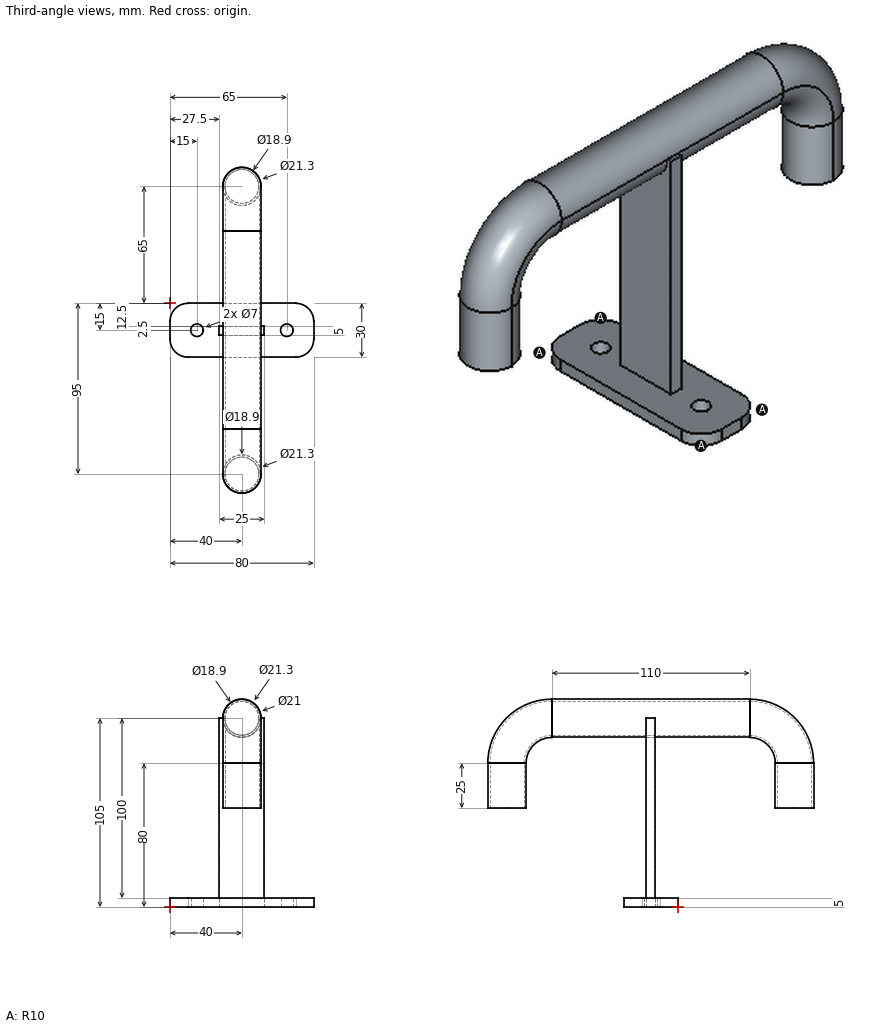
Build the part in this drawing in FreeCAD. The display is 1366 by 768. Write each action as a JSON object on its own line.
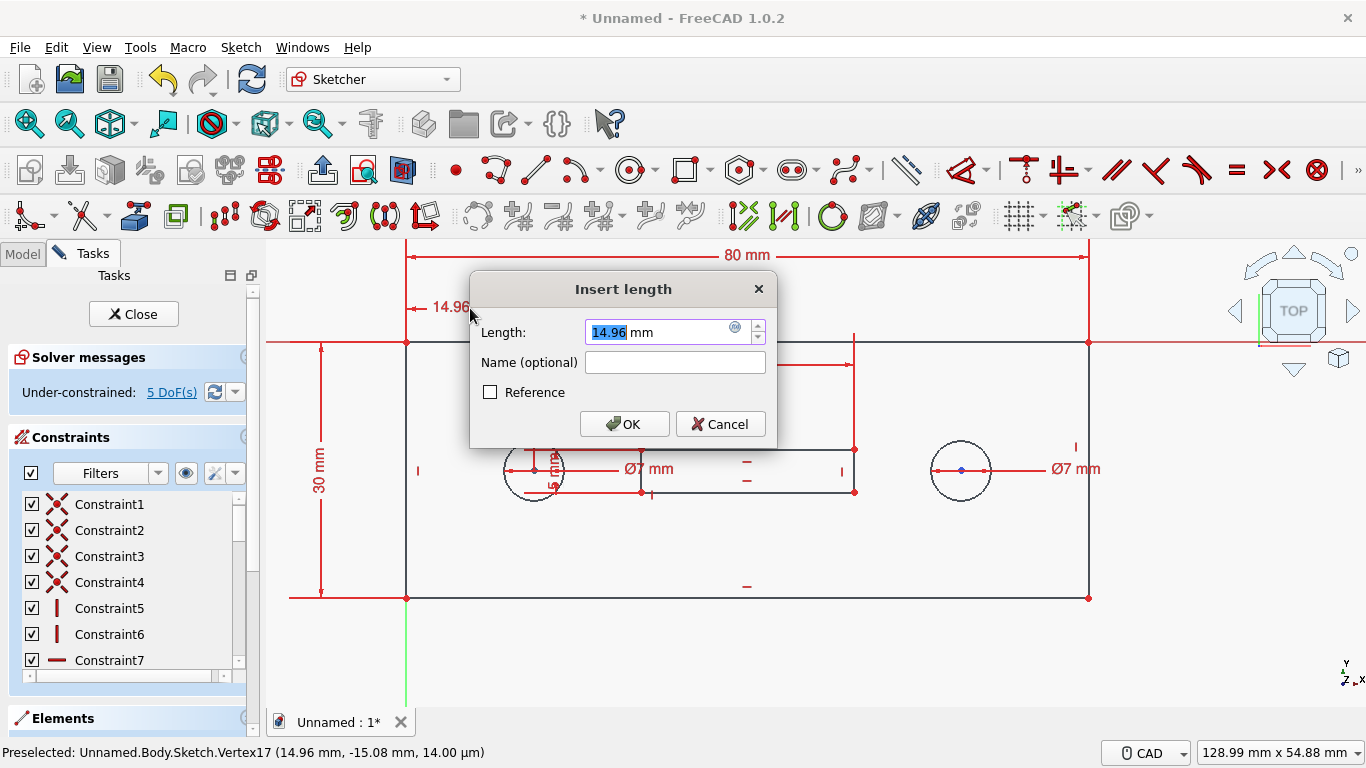
{"action": "type", "text": "15"}
{"action": "key", "text": "Return"}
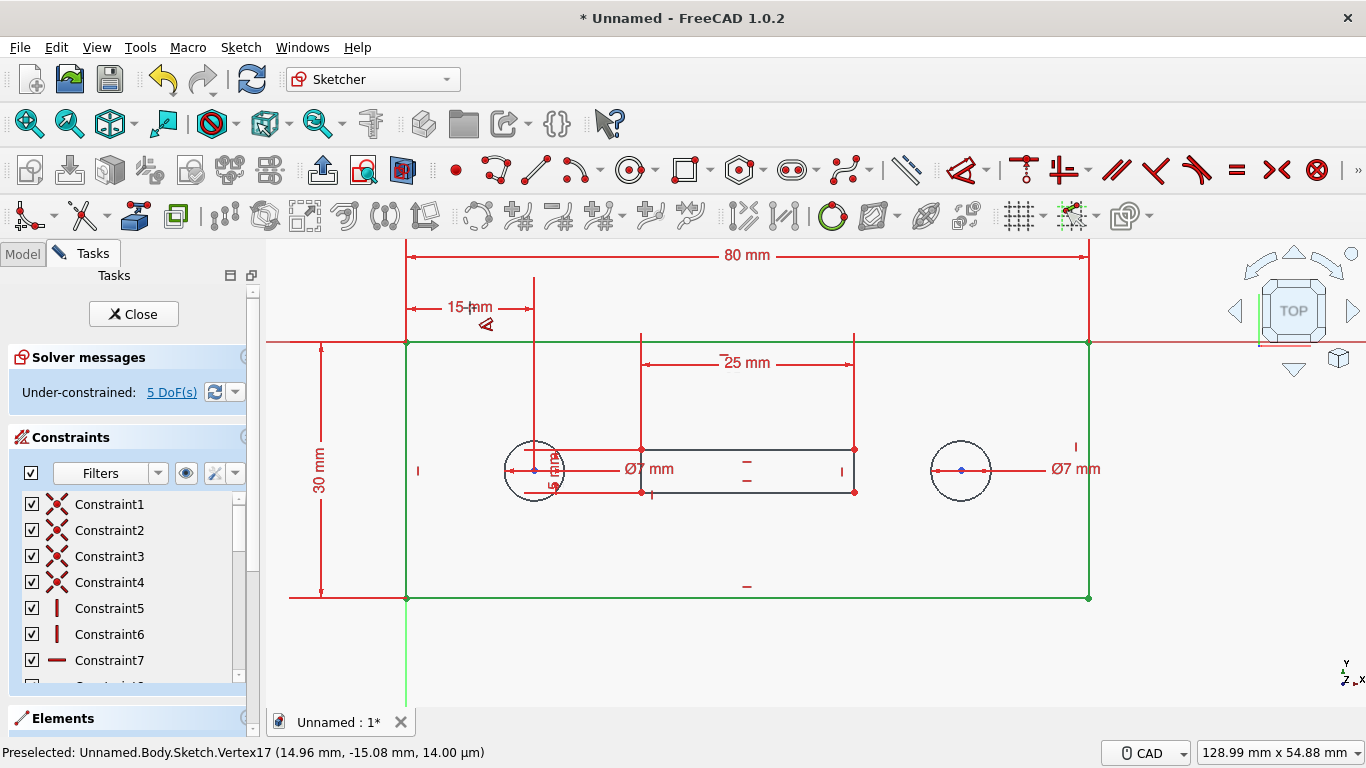
{"action": "left_click", "coordinate": [534, 471]}
{"action": "left_click", "coordinate": [372, 407]}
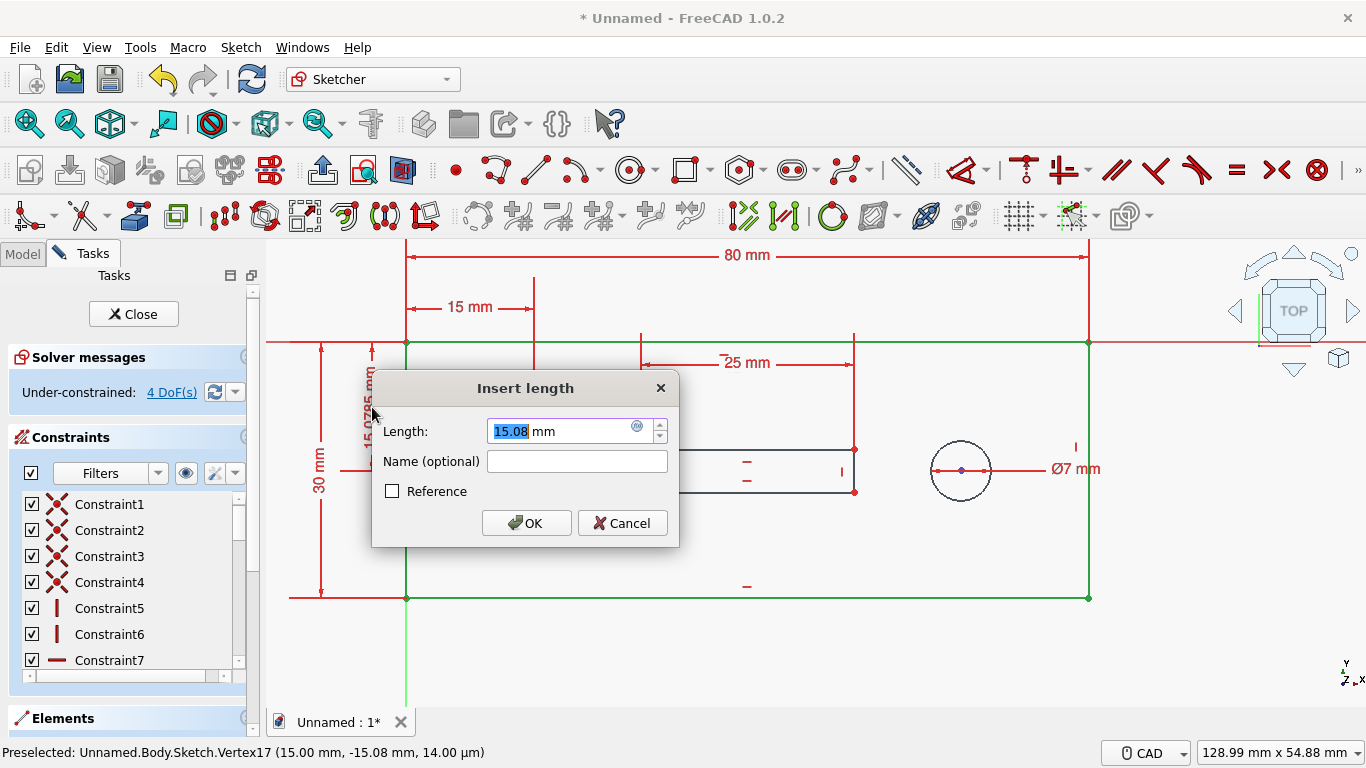
{"action": "type", "text": "15"}
{"action": "key", "text": "Return"}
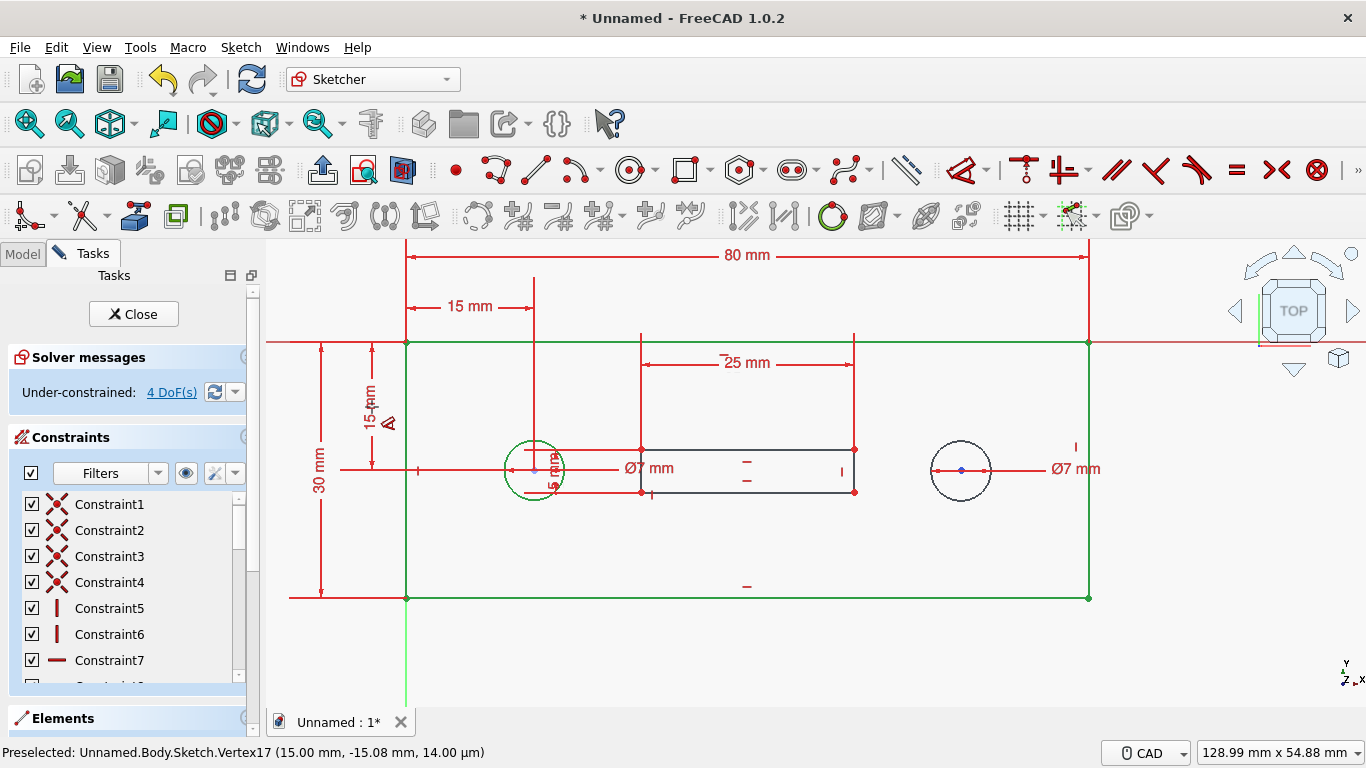
{"action": "left_click", "coordinate": [961, 471]}
{"action": "left_click", "coordinate": [684, 308]}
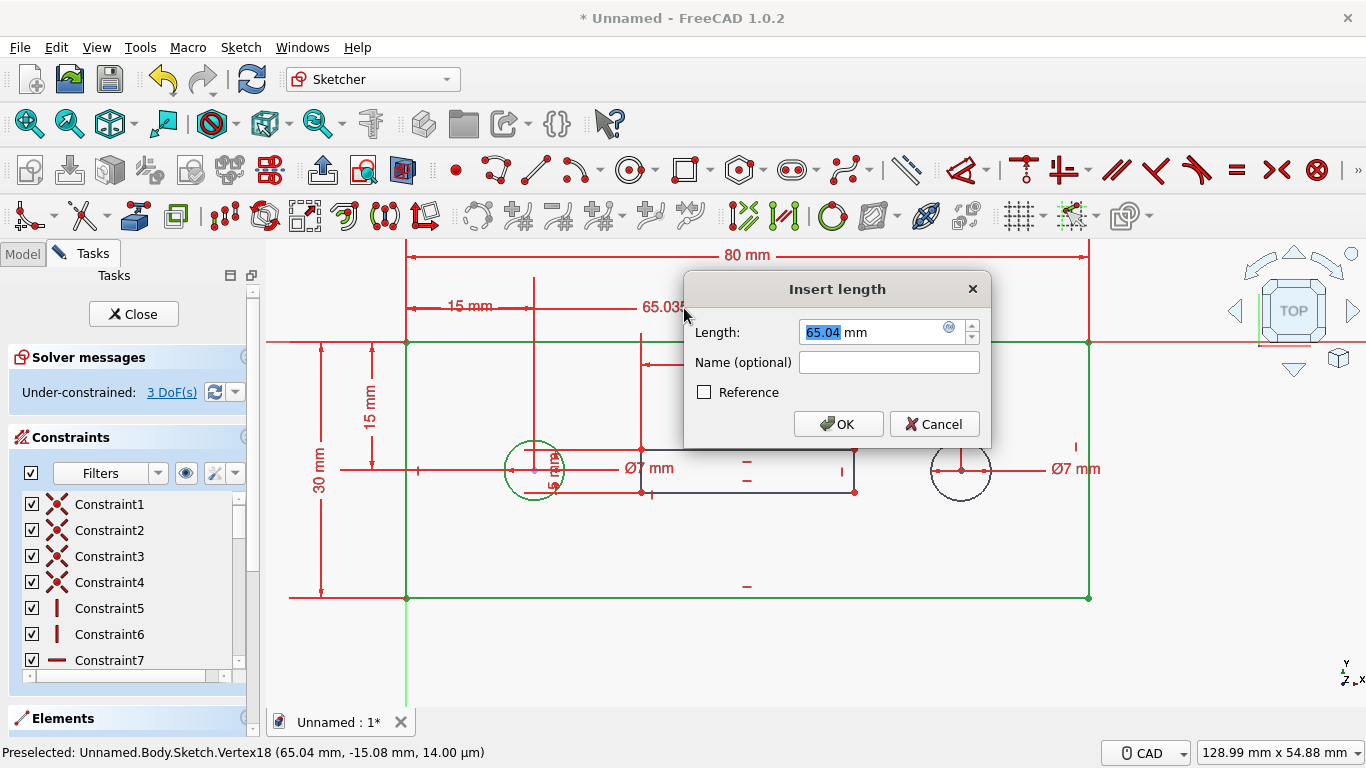
{"action": "type", "text": "65"}
{"action": "key", "text": "Return"}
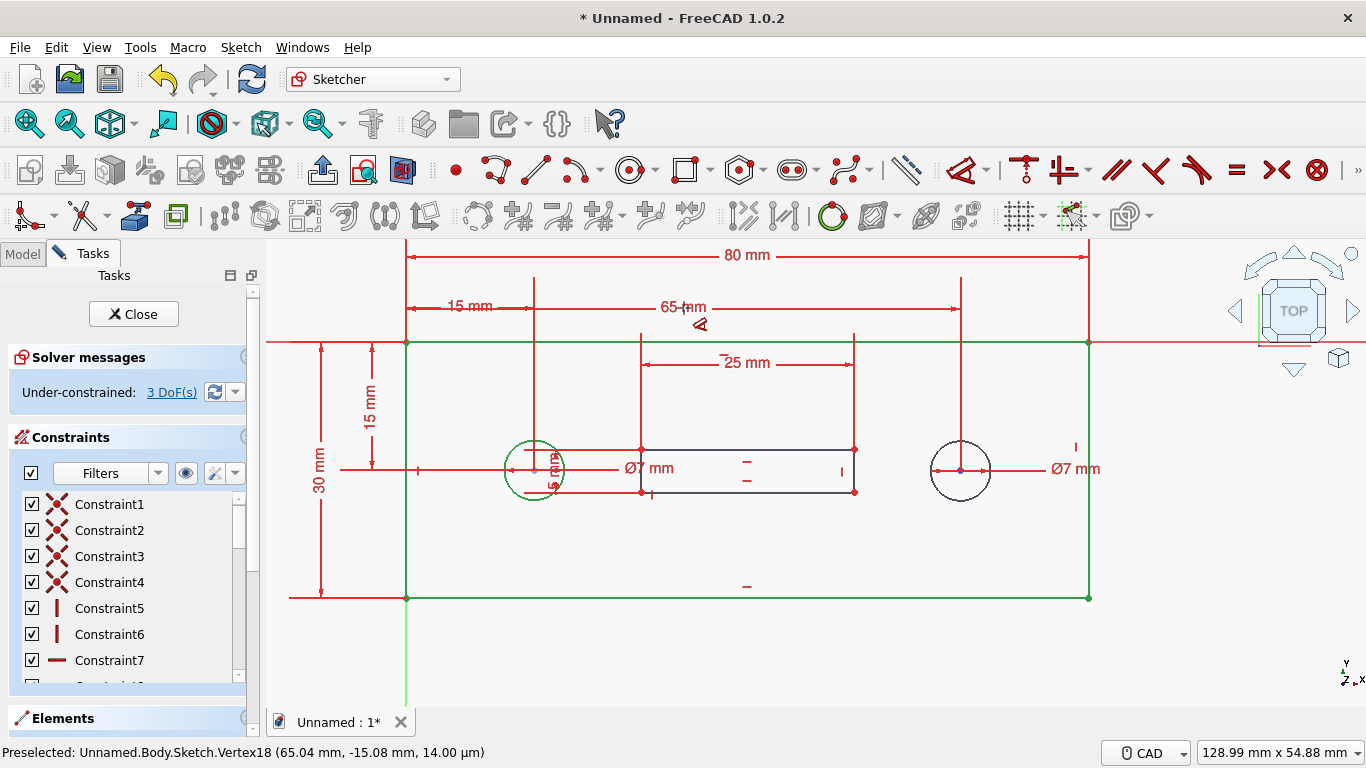
{"action": "left_click", "coordinate": [961, 471]}
{"action": "left_click", "coordinate": [372, 377]}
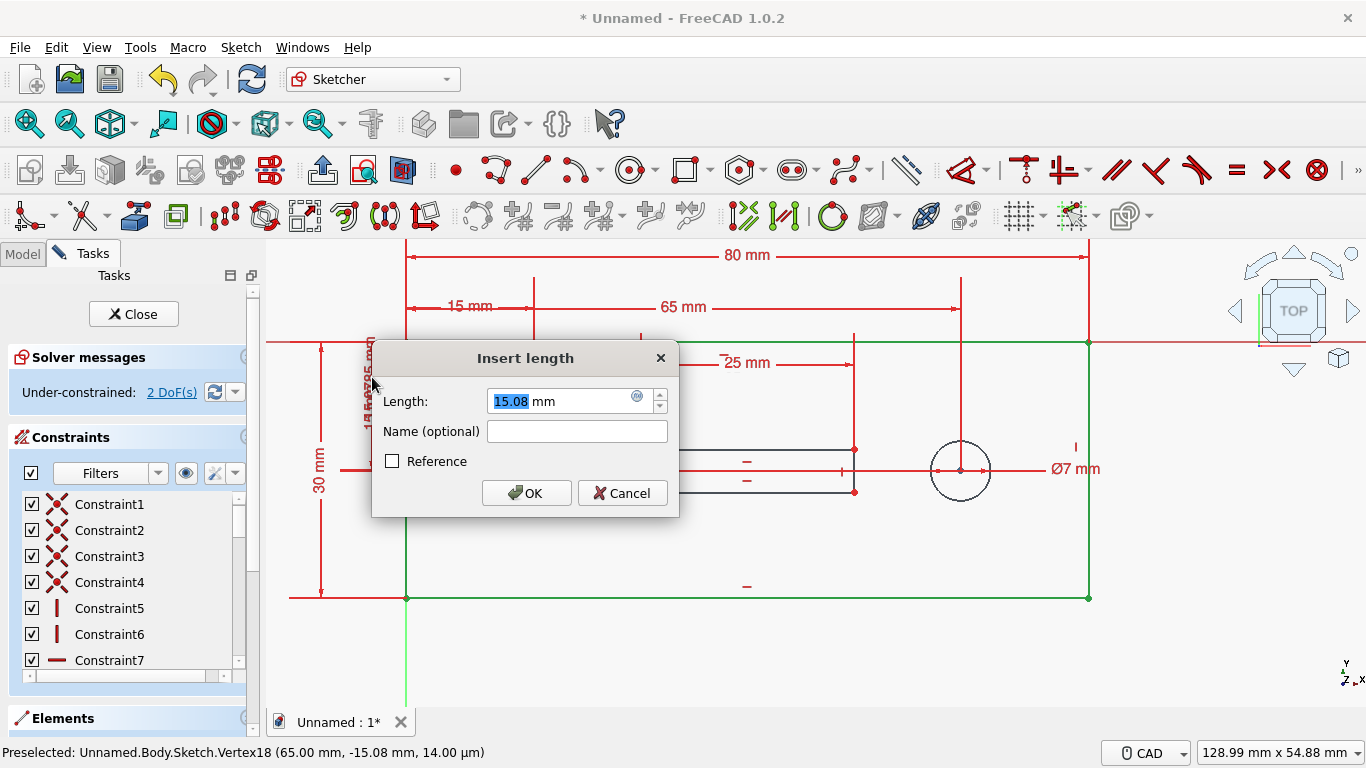
{"action": "type", "text": "15"}
{"action": "key", "text": "Return"}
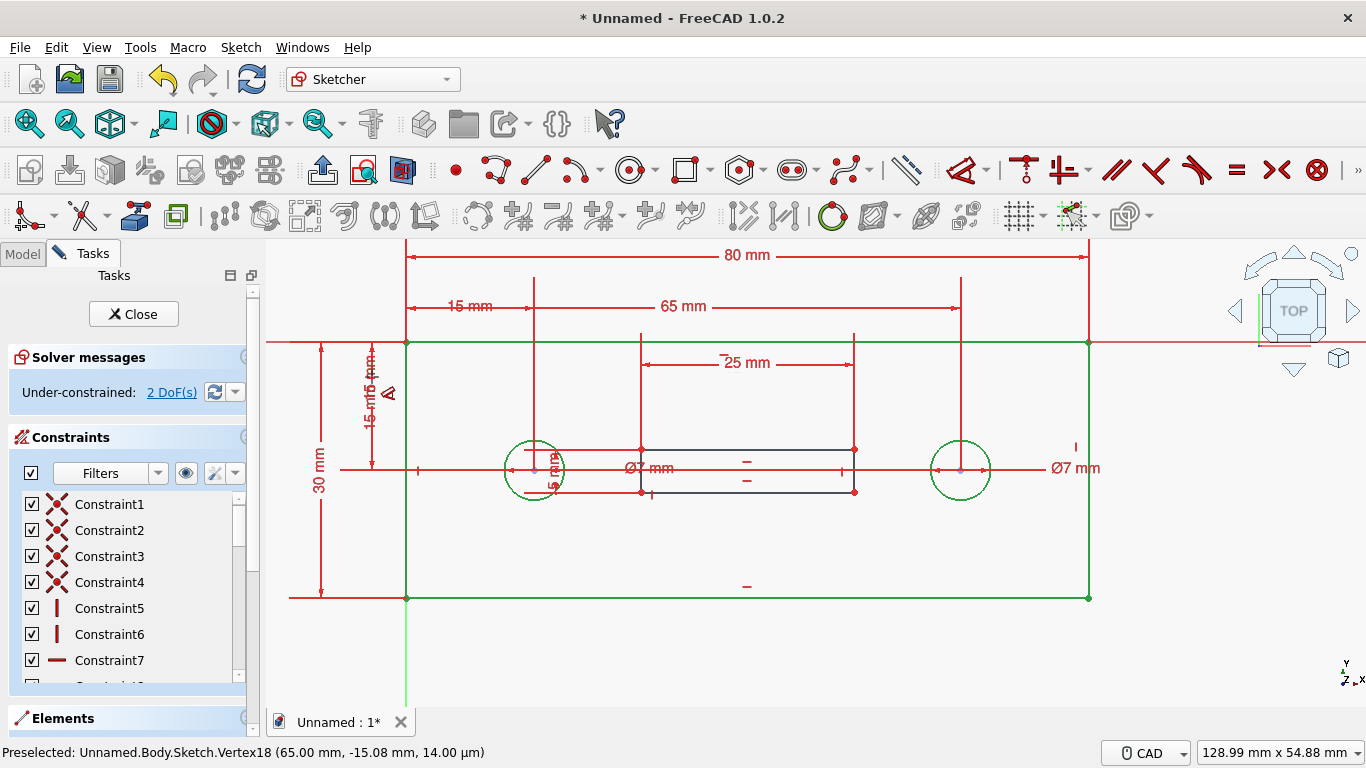
{"action": "scroll", "coordinate": [641, 450], "scroll_direction": "up", "scroll_amount": 4}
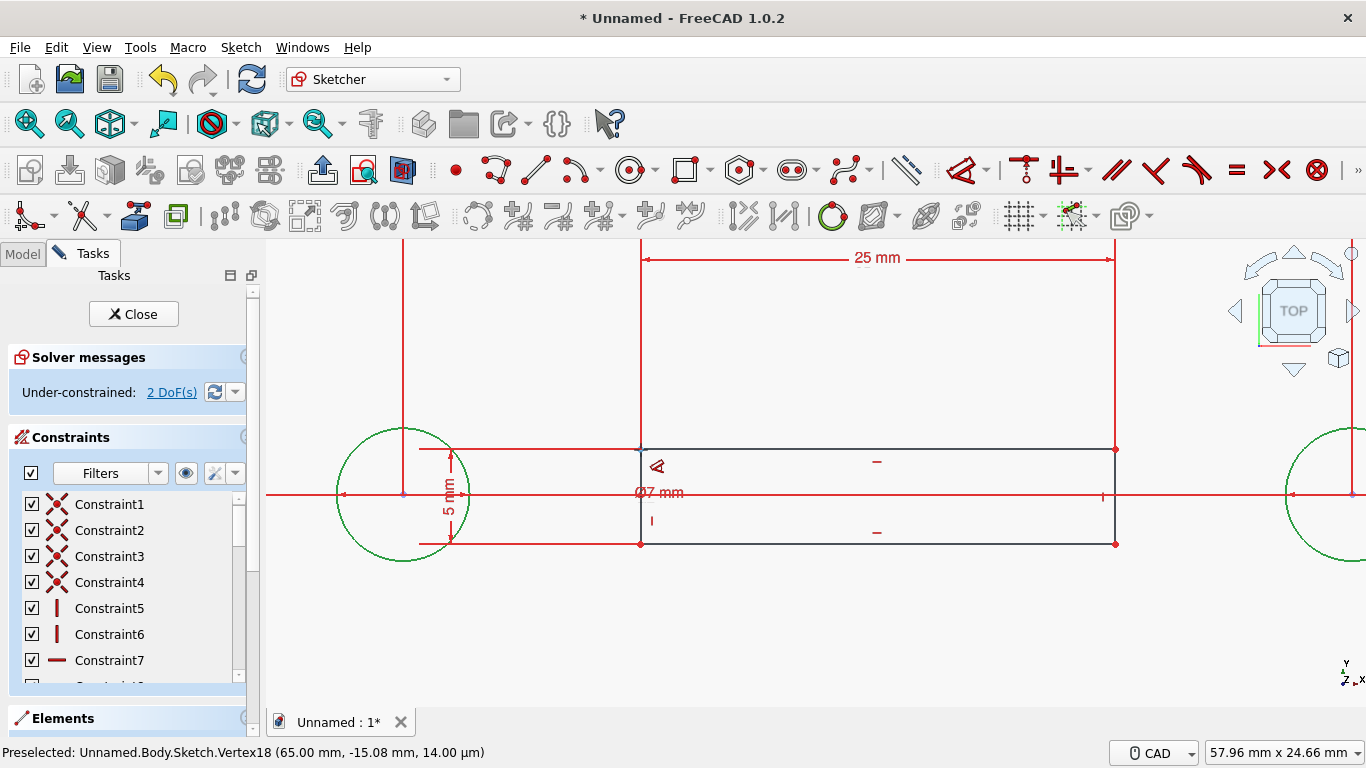
{"action": "left_click", "coordinate": [641, 449]}